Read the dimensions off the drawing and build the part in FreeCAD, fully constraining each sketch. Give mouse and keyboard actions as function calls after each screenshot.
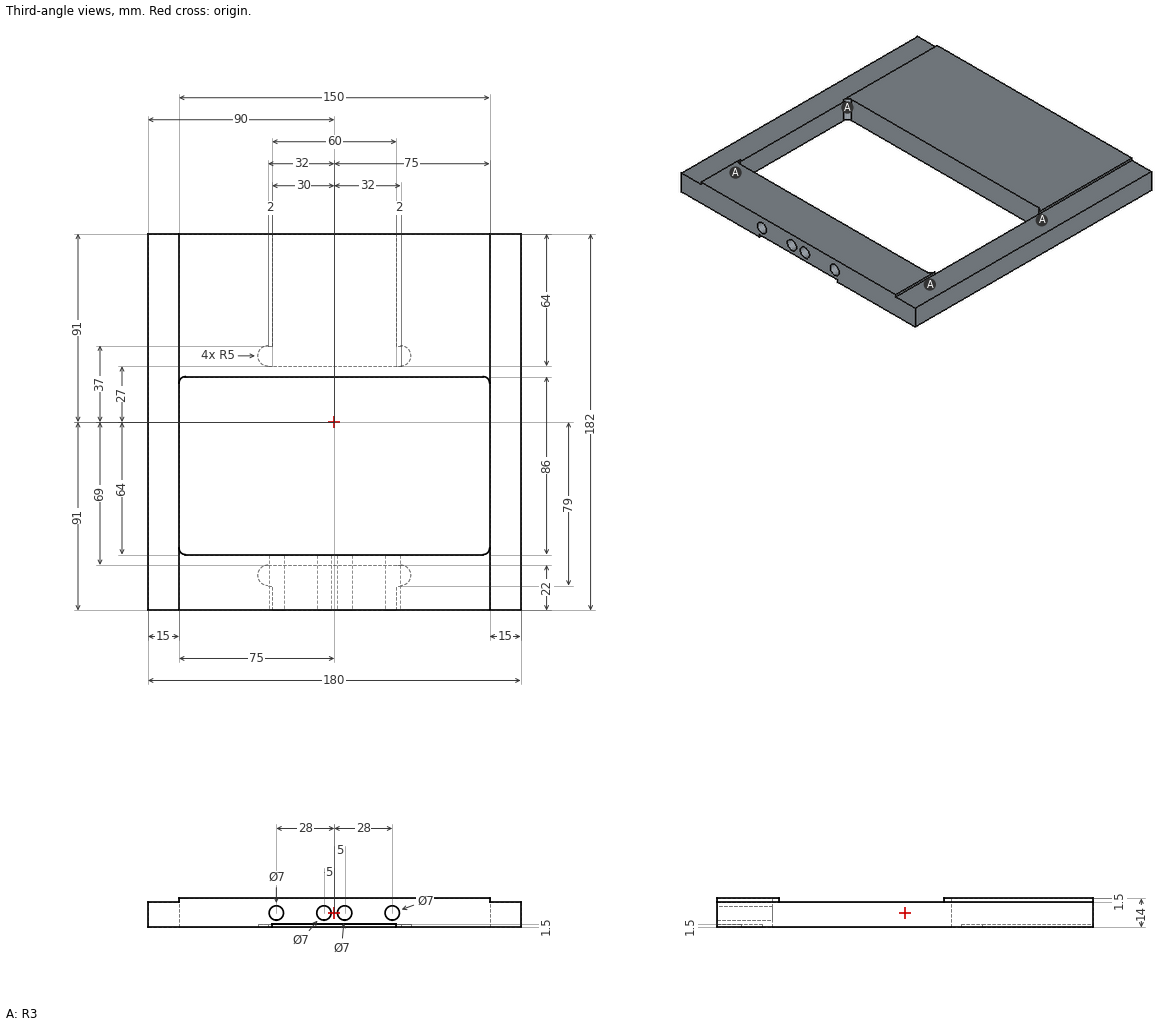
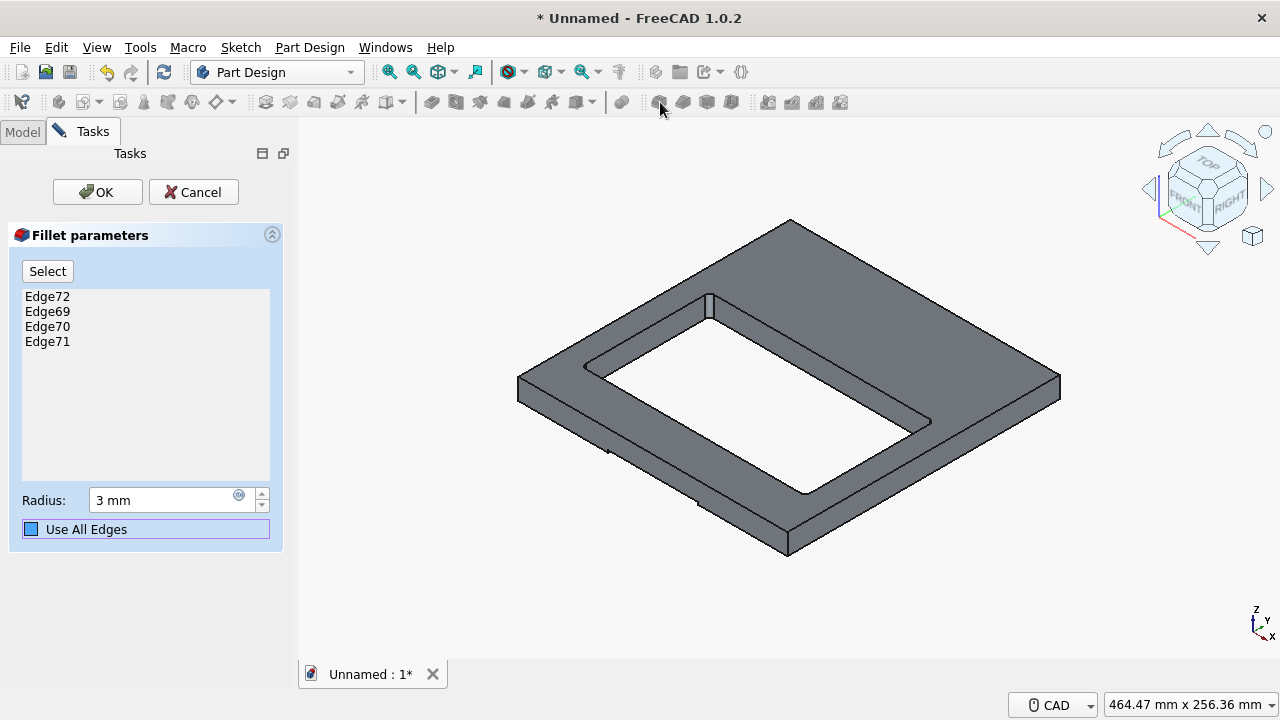
click(98, 192)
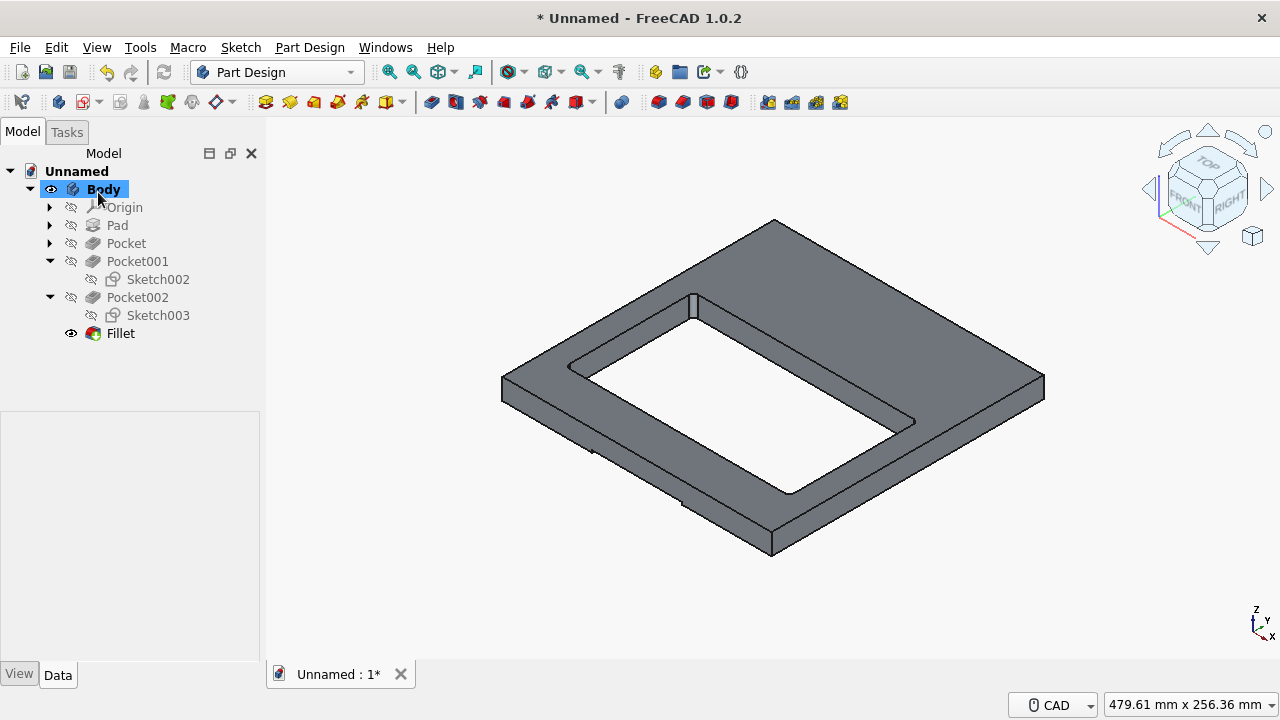
click(752, 532)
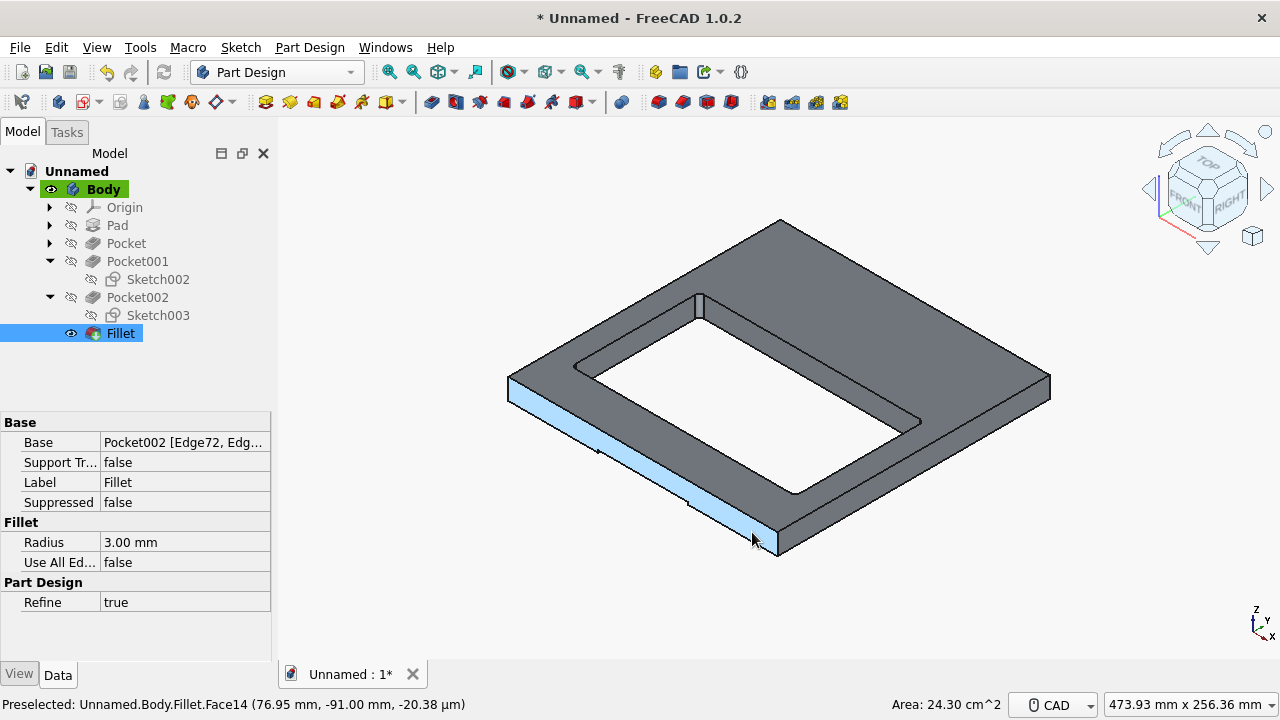
click(84, 102)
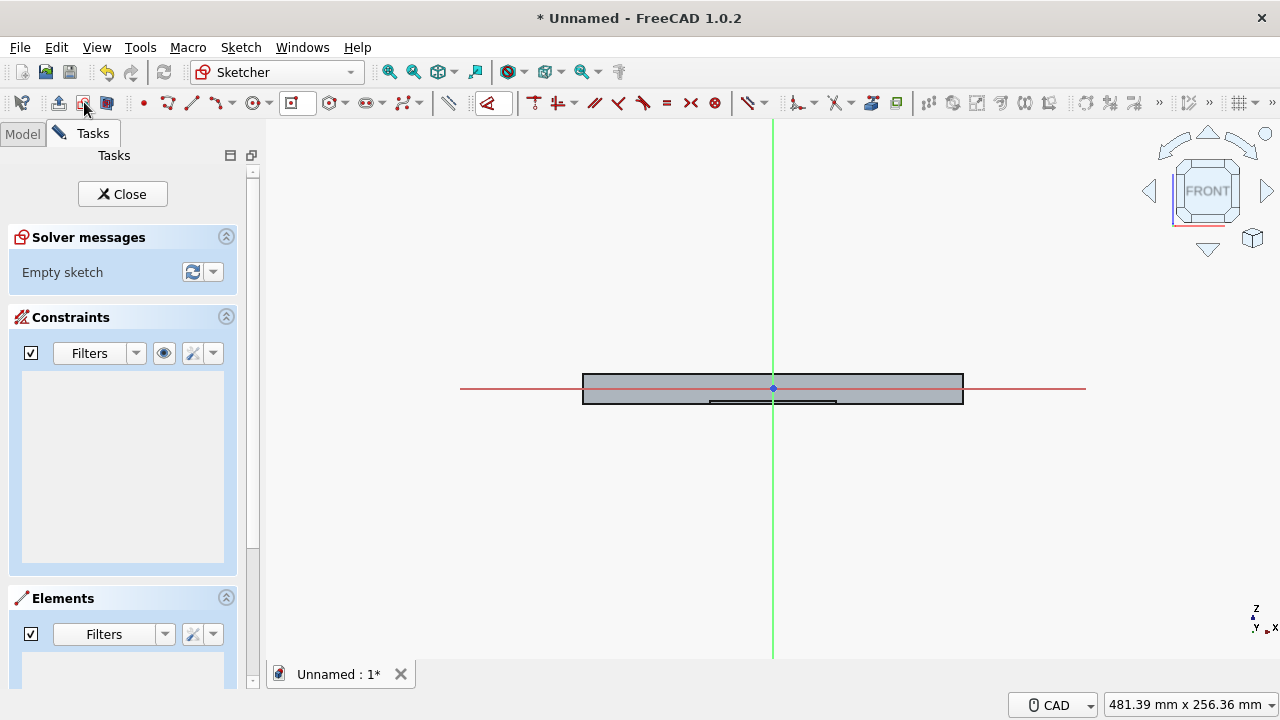
scroll(715, 389, up, 15)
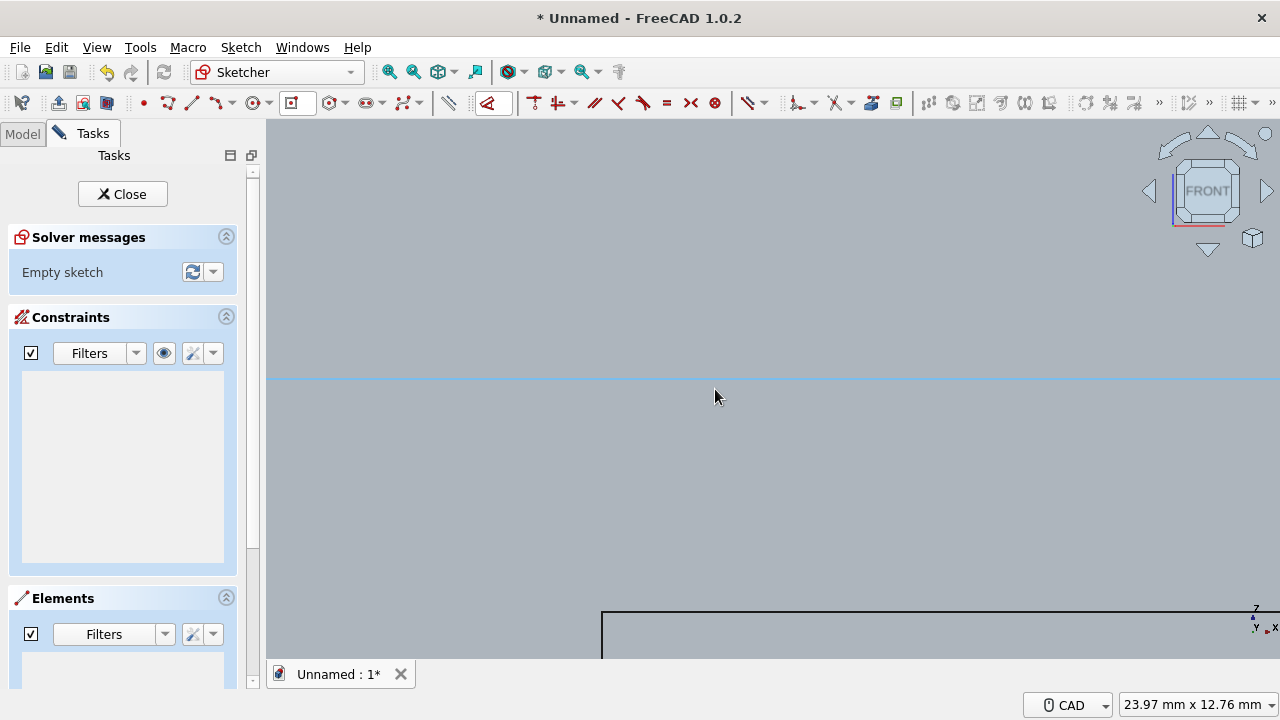
key(g)
key(c)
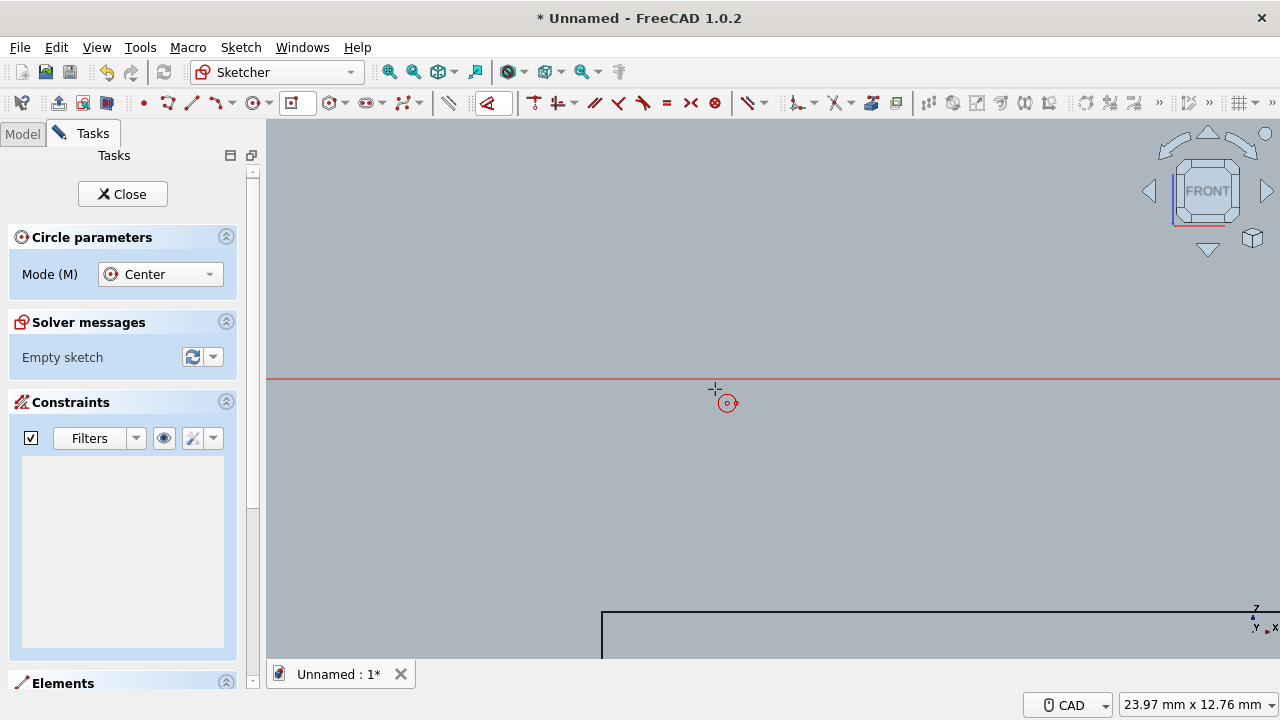
click(687, 379)
move(792, 275)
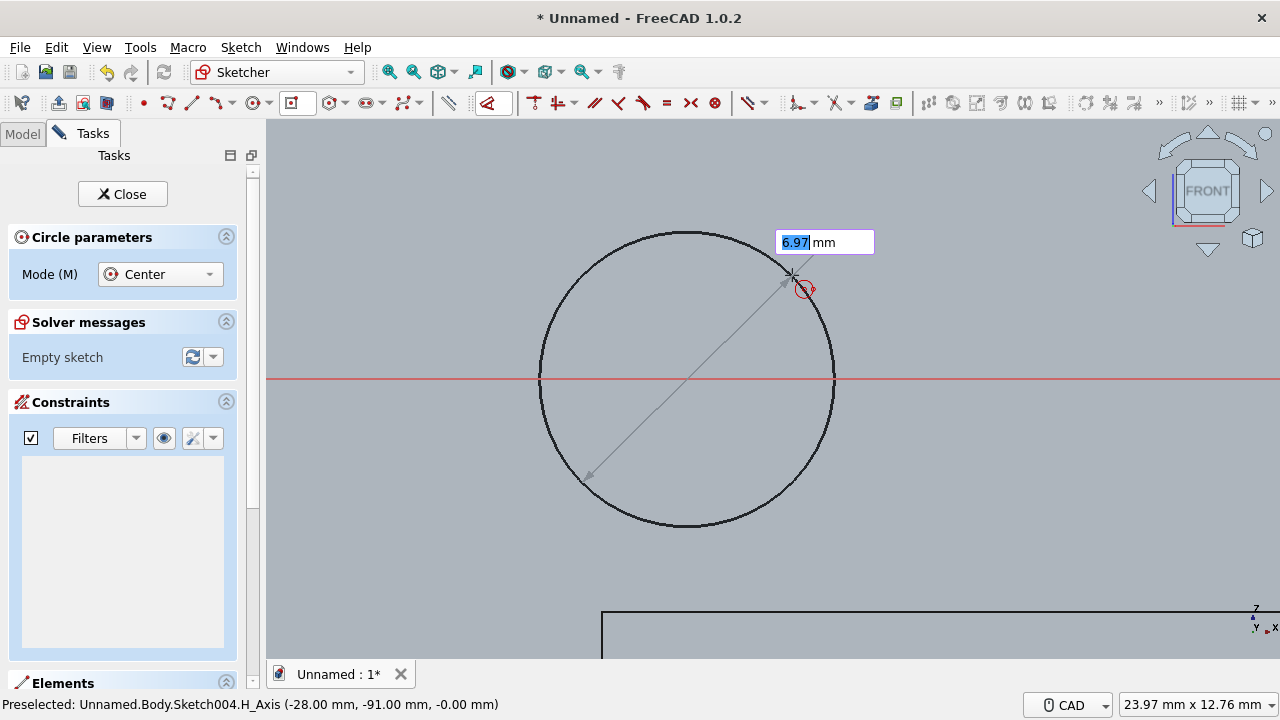
text(7)
key(Return)
key(Escape)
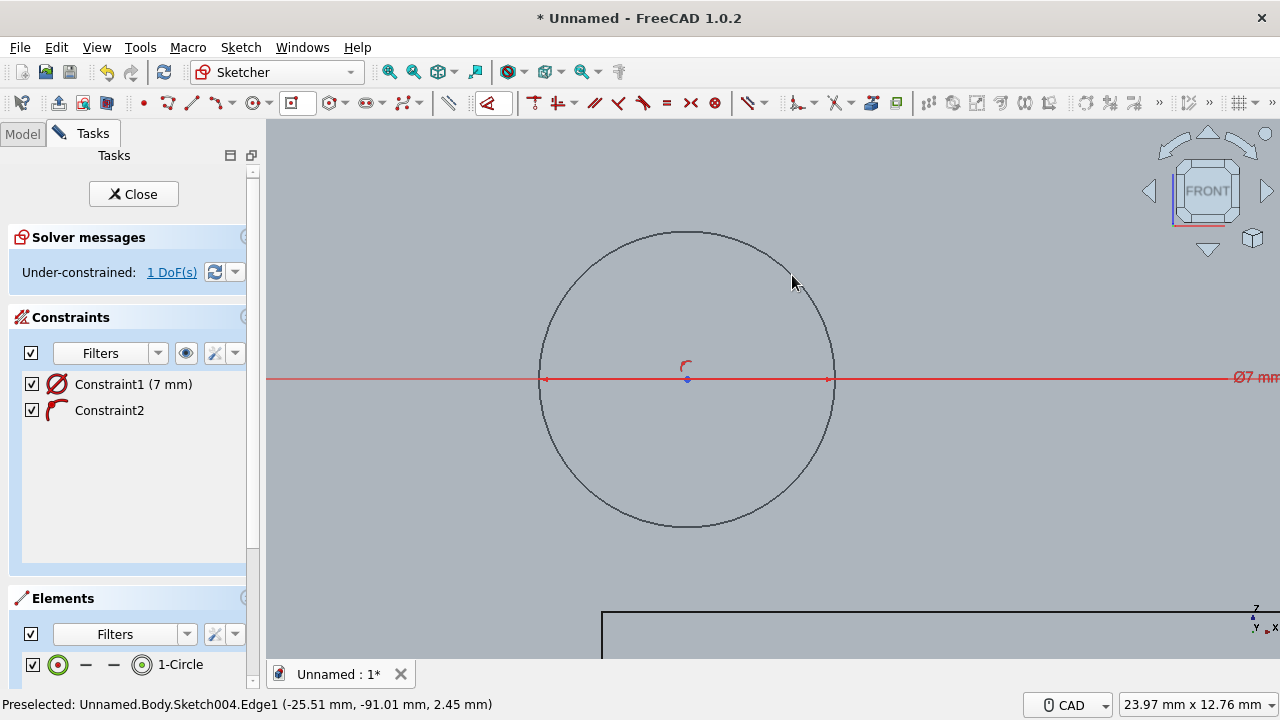
click(687, 379)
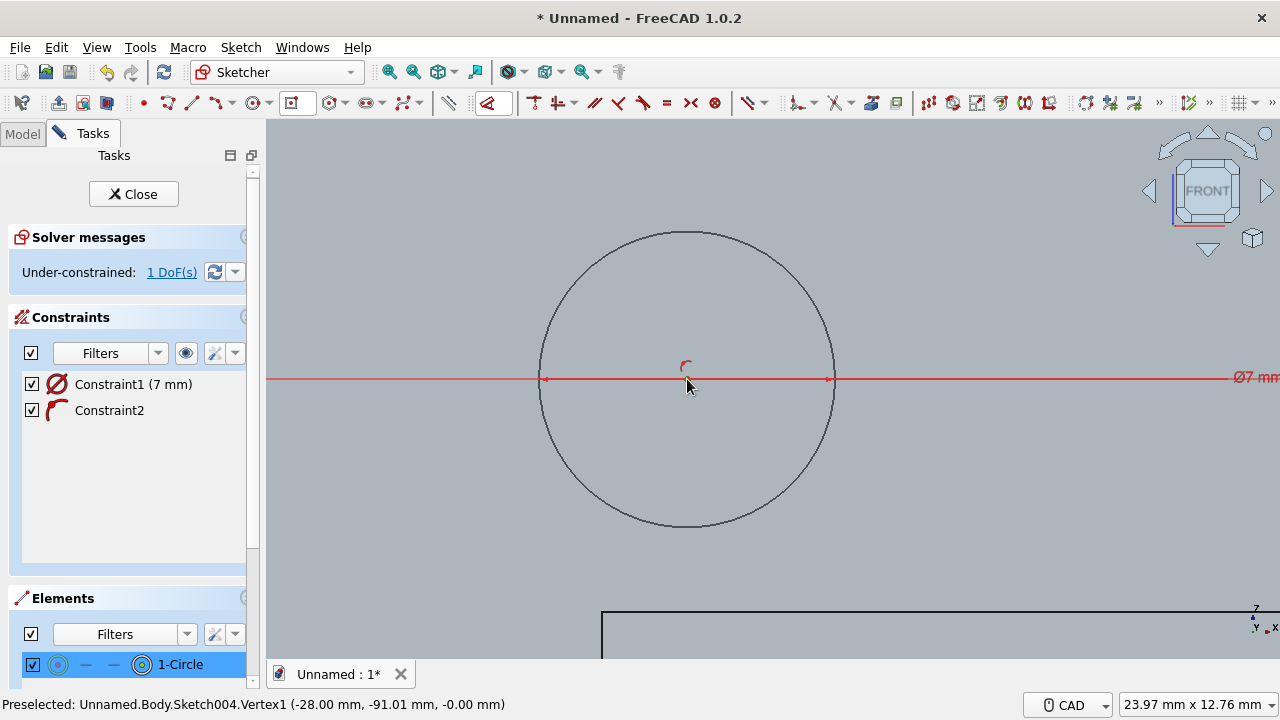
key(l)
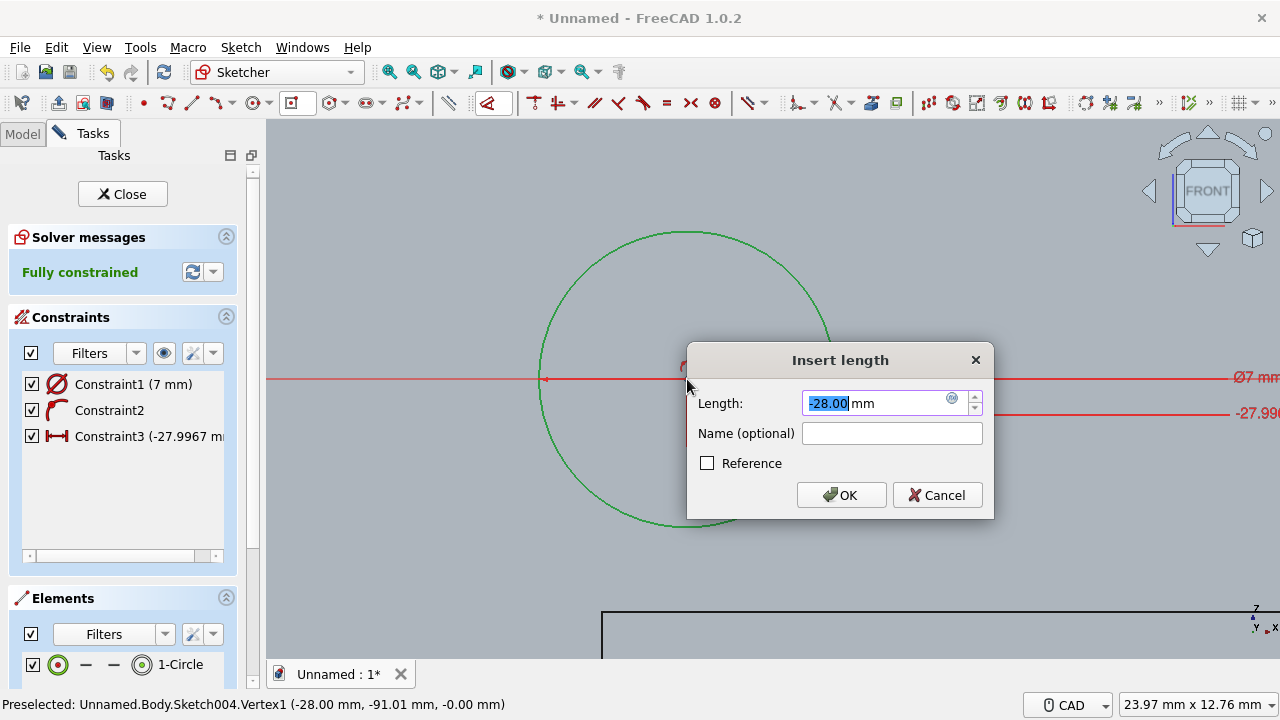
text(-28)
key(Return)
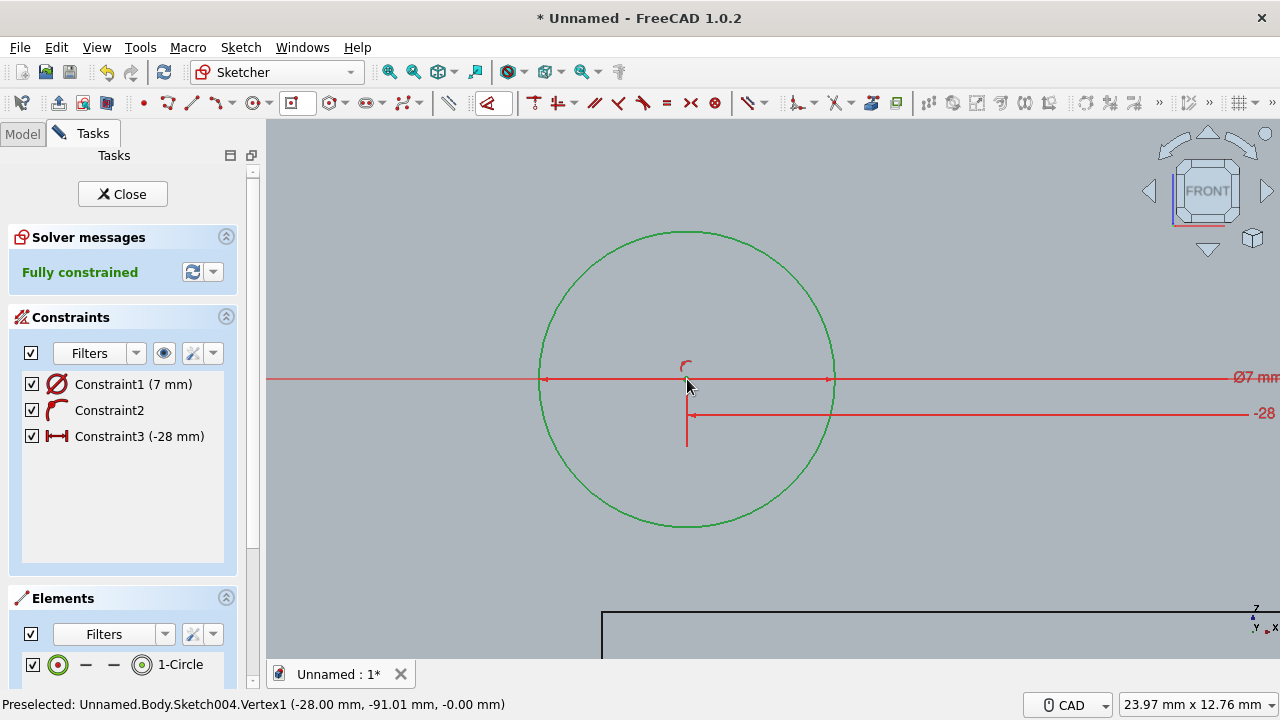
click(123, 194)